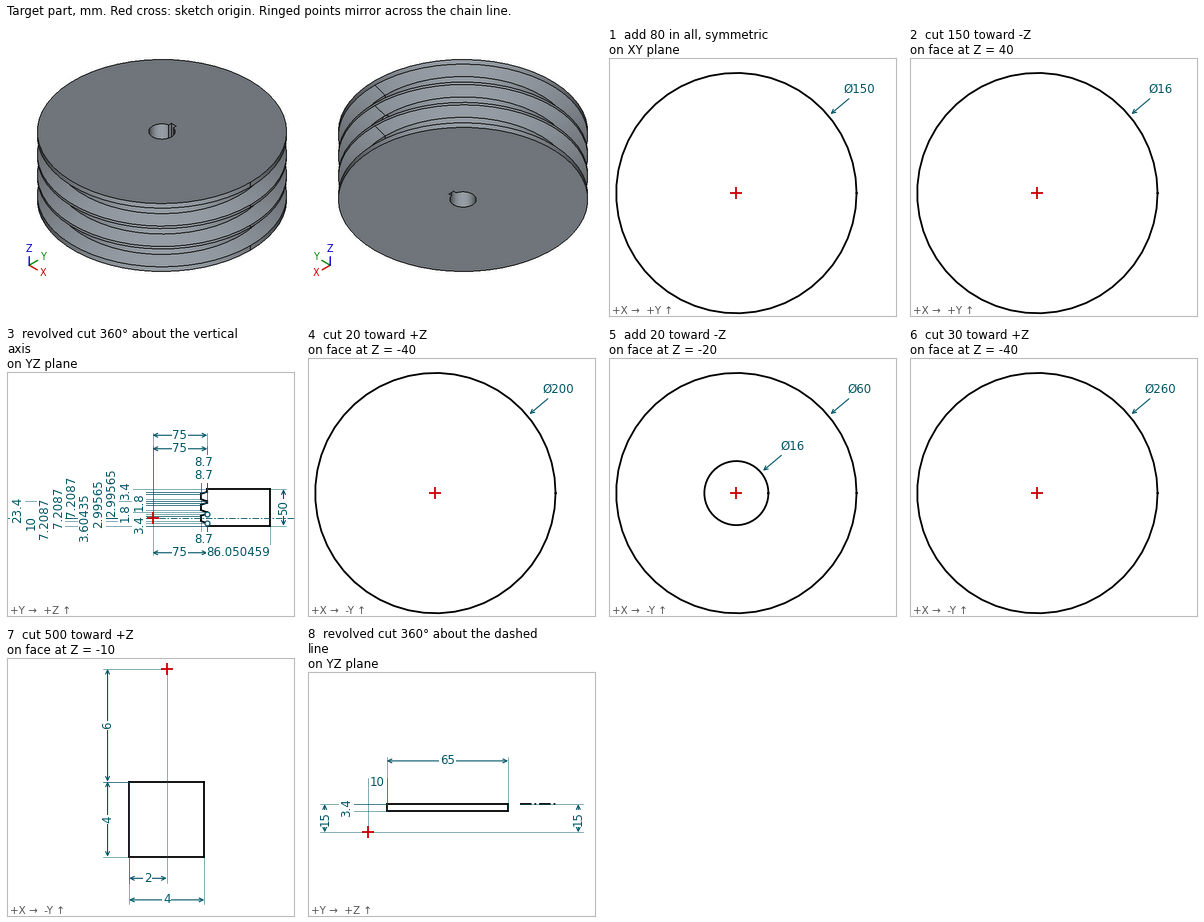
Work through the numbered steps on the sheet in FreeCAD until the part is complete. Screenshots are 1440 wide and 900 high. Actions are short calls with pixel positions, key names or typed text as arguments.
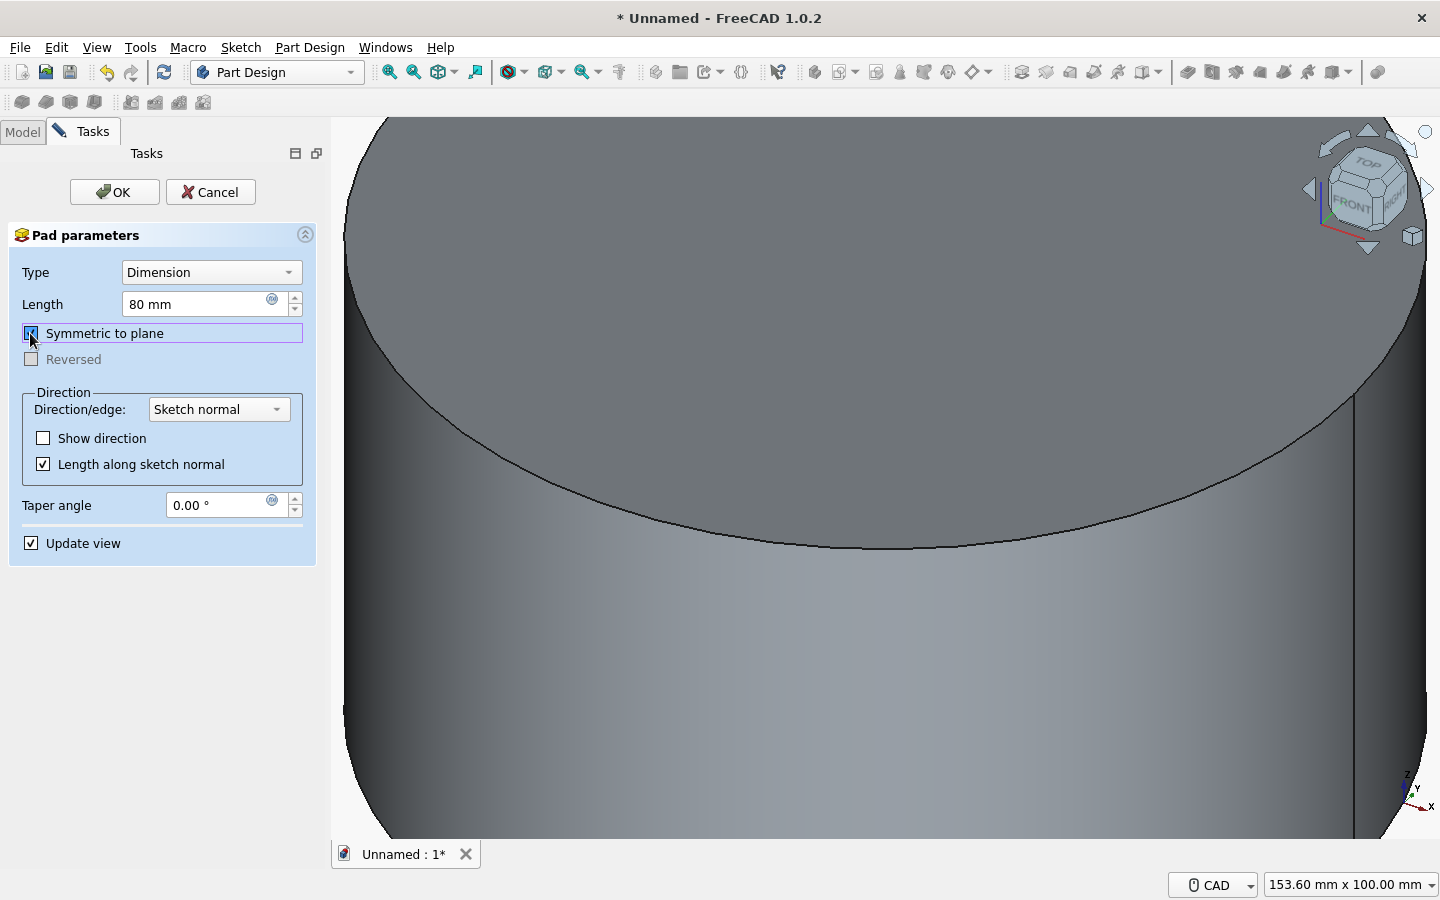
click(115, 192)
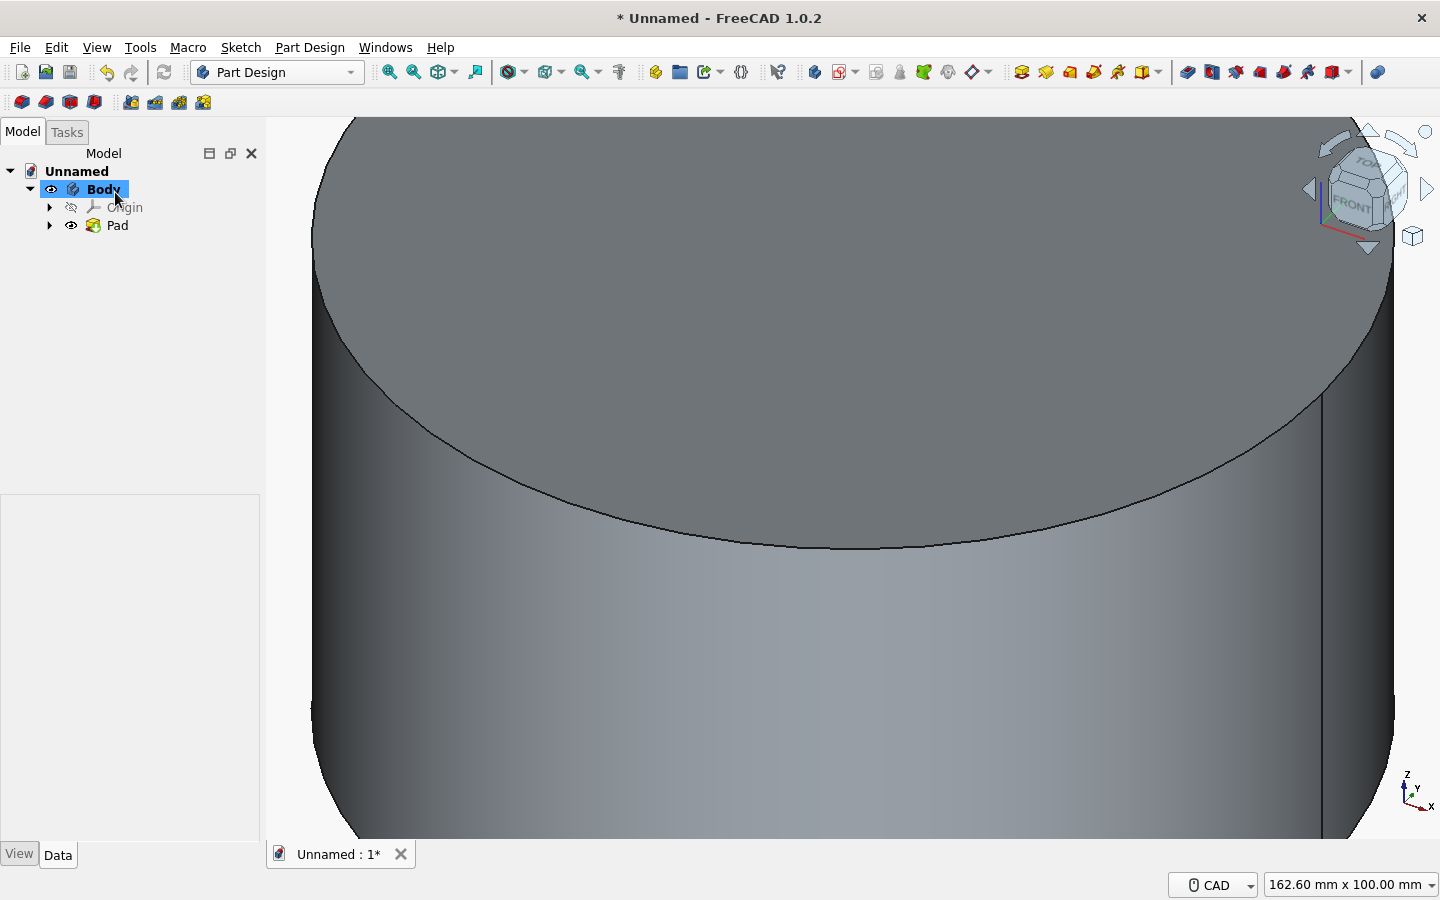
key(v)
key(f)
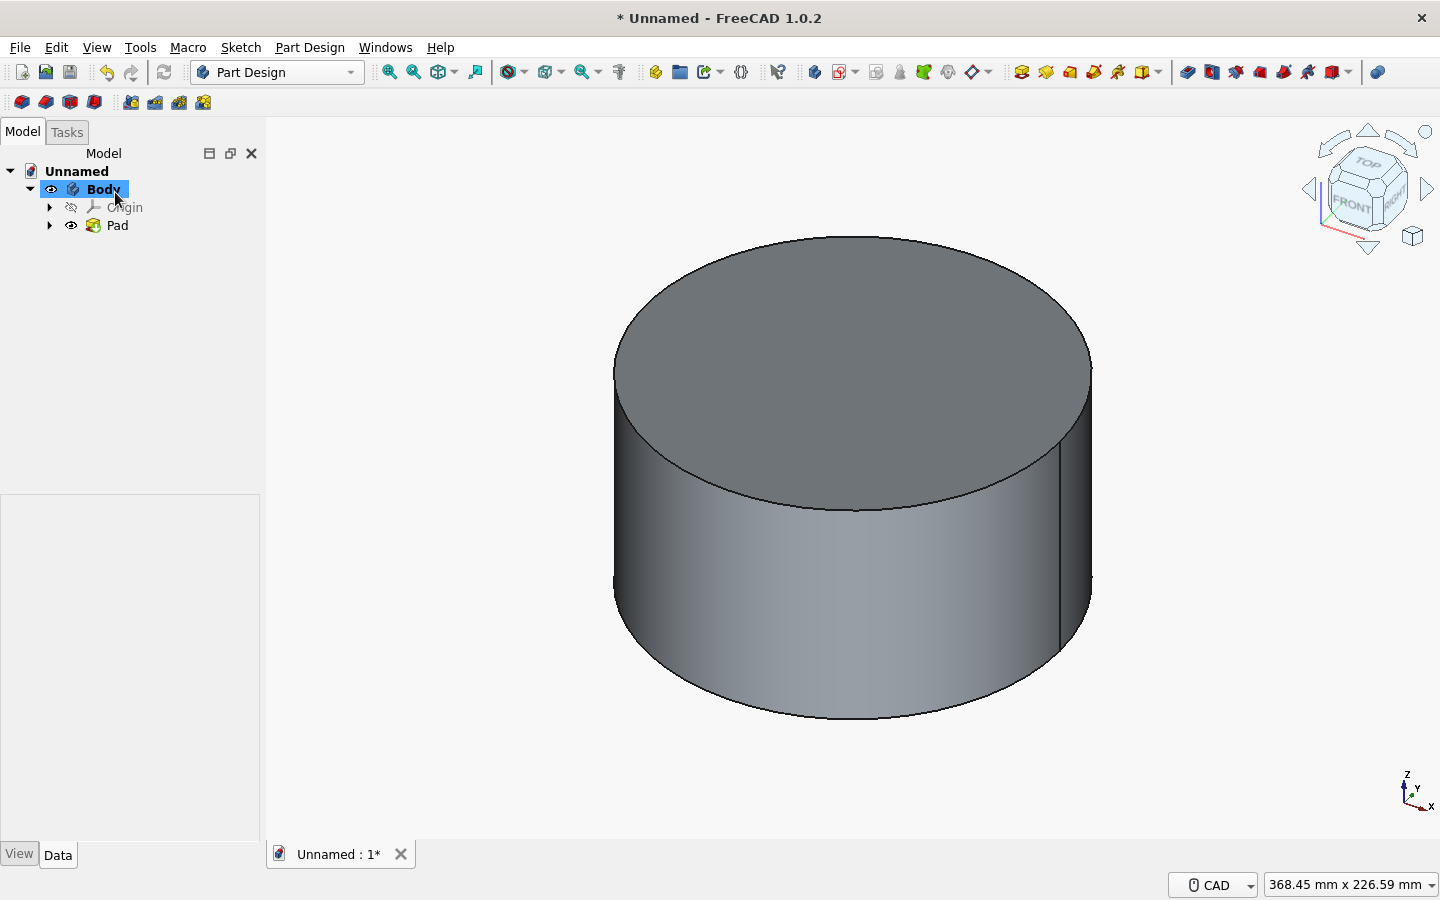
click(853, 373)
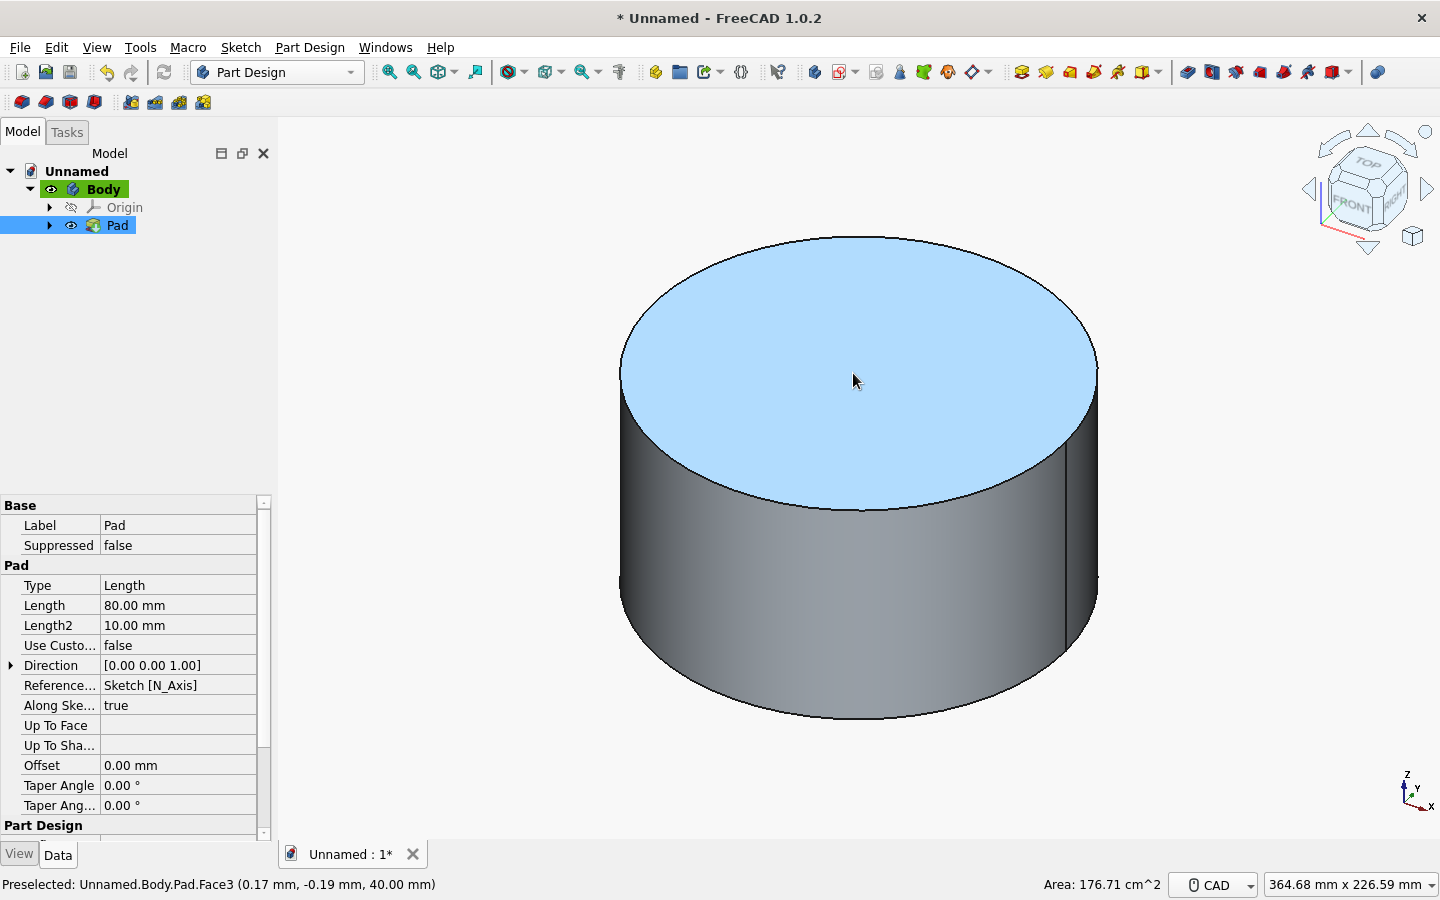
click(840, 72)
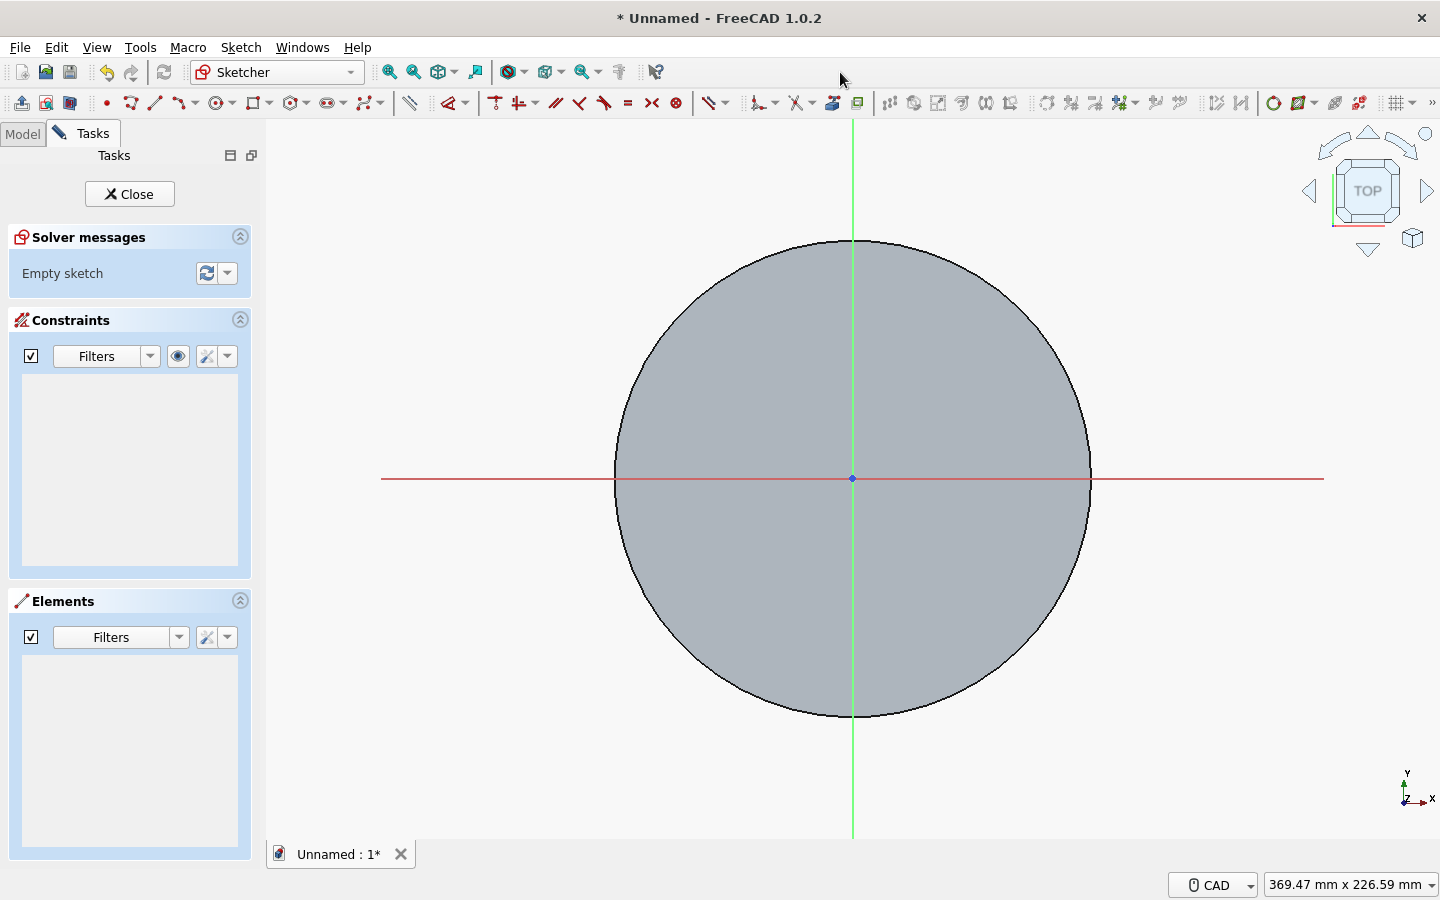
scroll(861, 479, up, 11)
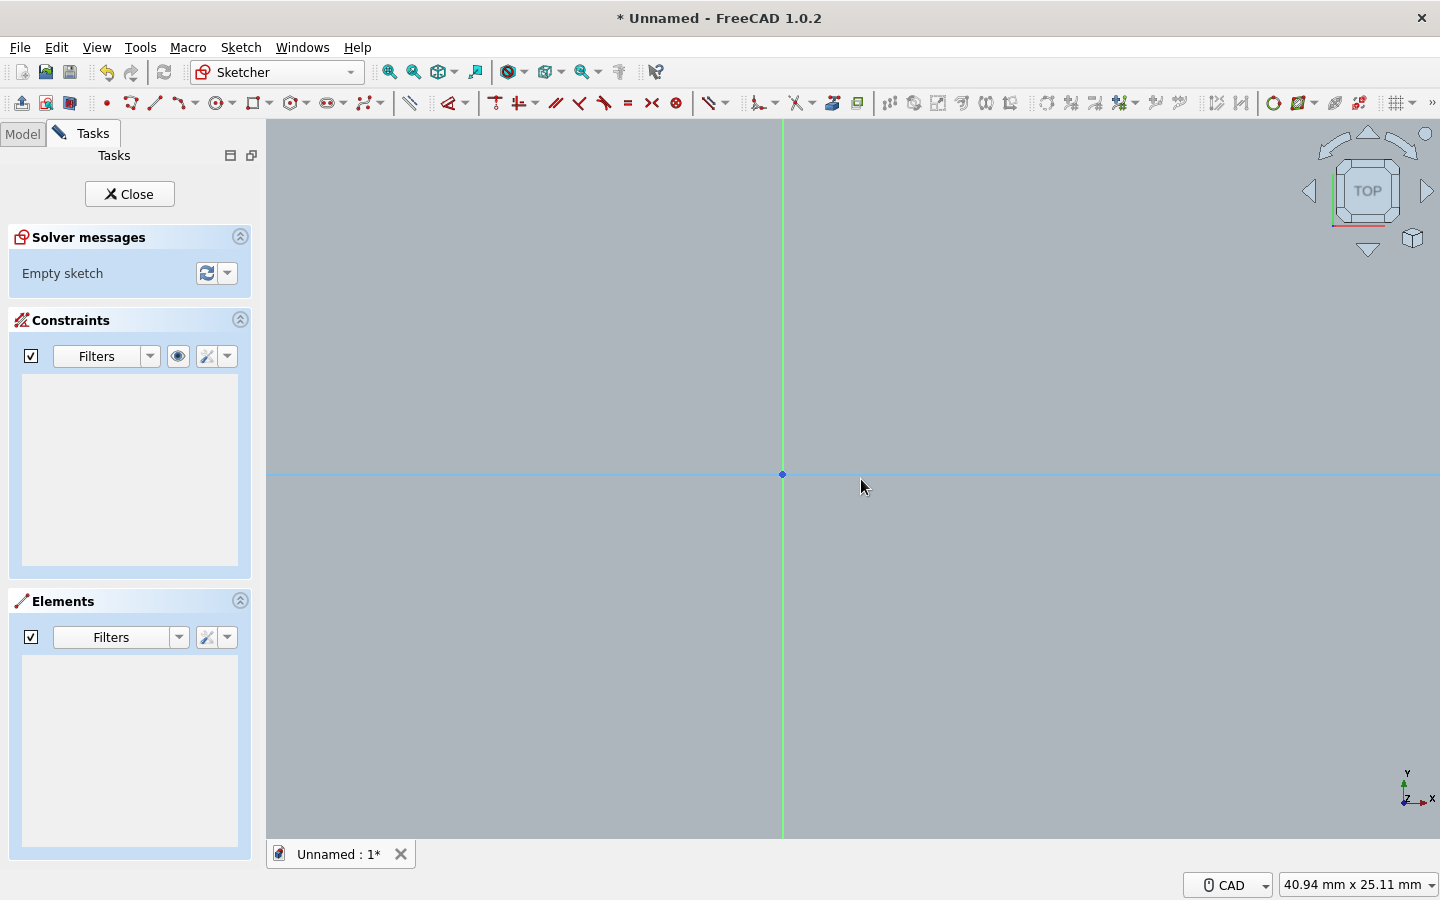
key(g)
key(c)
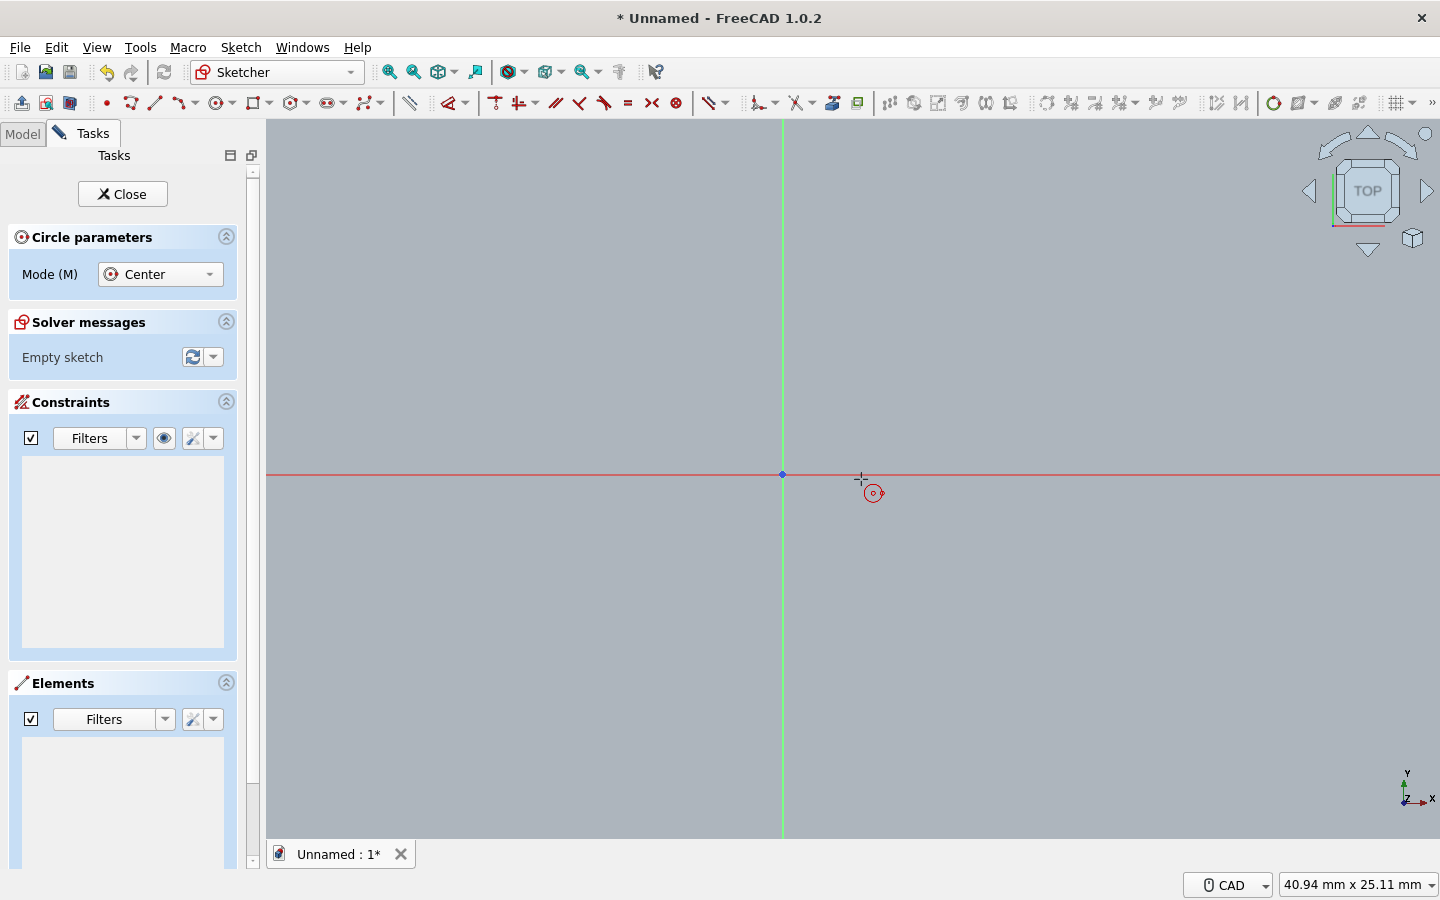
click(783, 475)
click(945, 313)
key(Escape)